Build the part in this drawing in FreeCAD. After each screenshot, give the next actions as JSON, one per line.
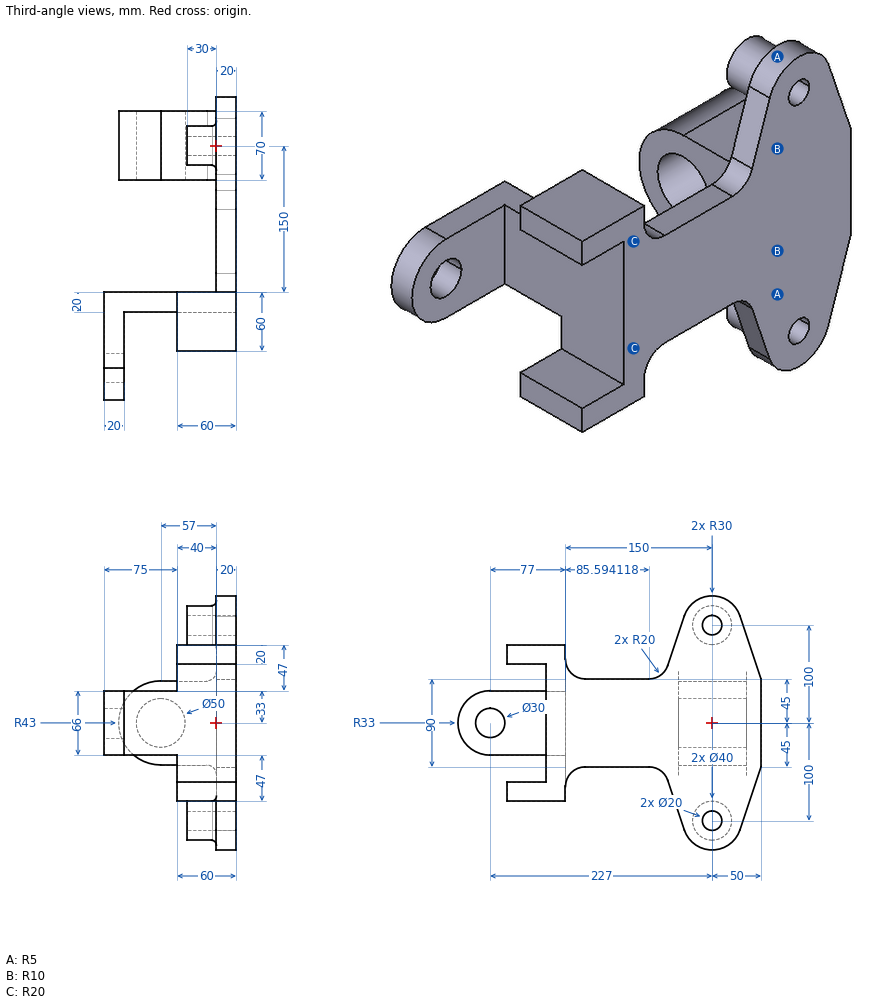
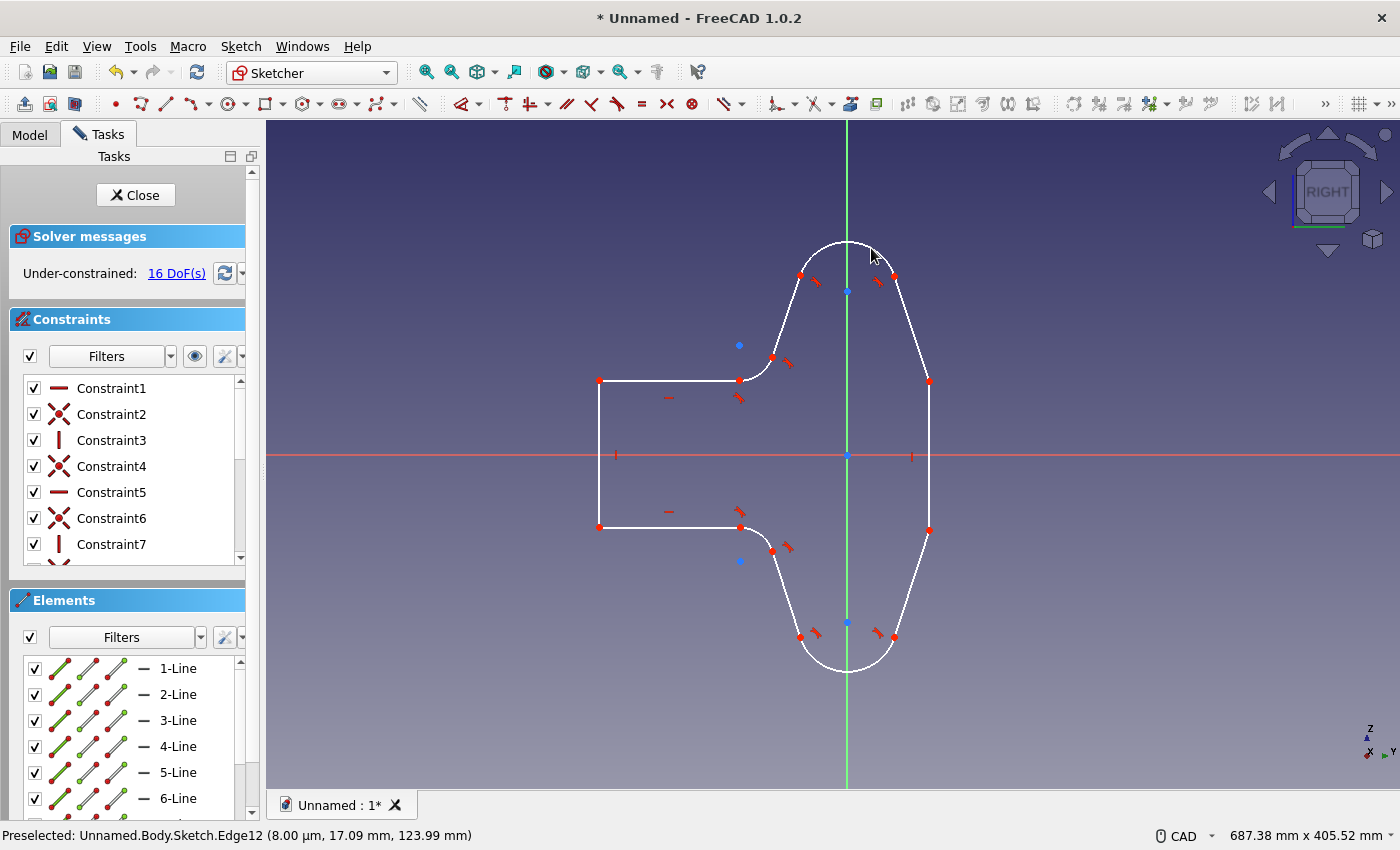
{"action": "left_click", "coordinate": [752, 378]}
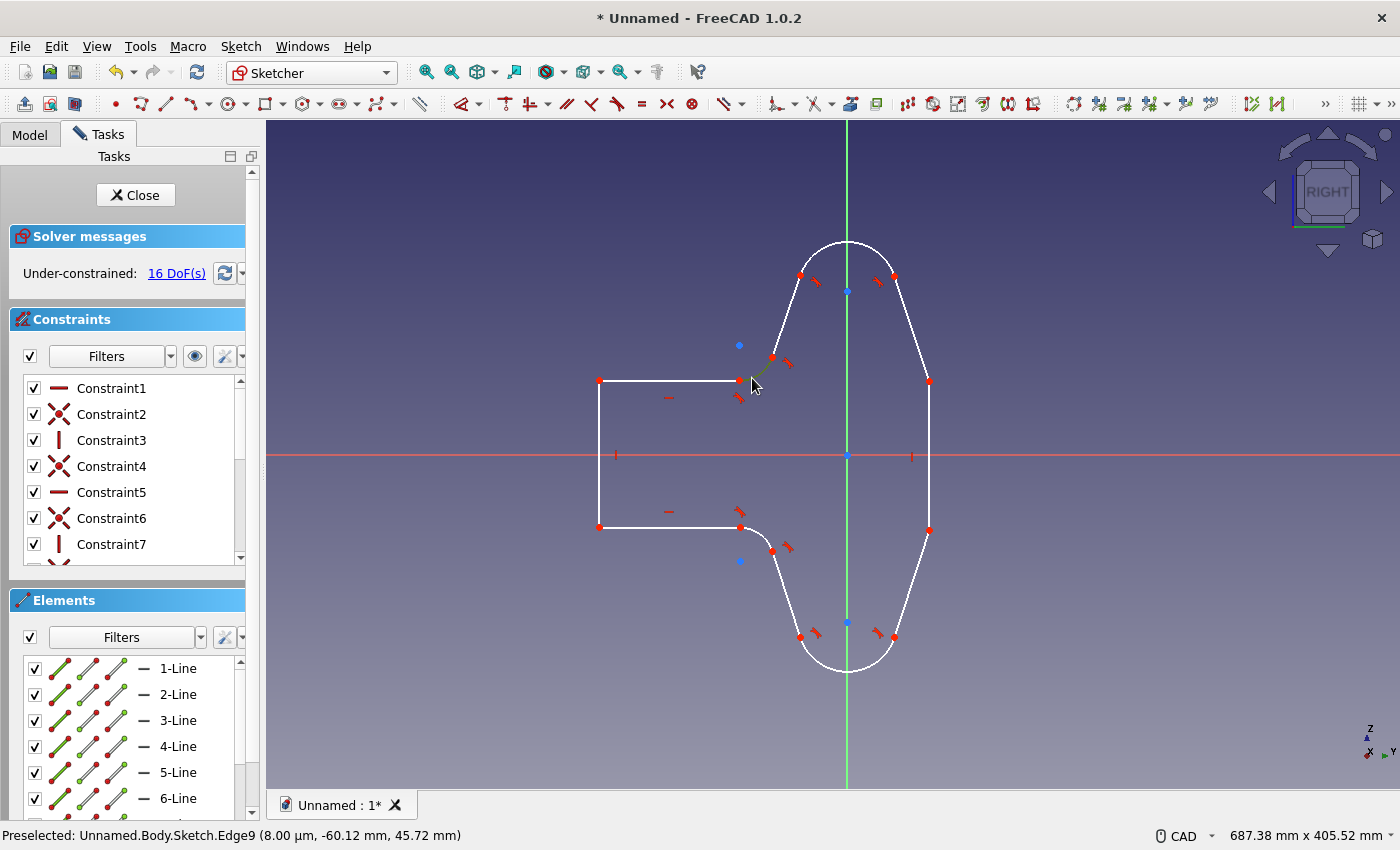
{"action": "left_click", "coordinate": [766, 540]}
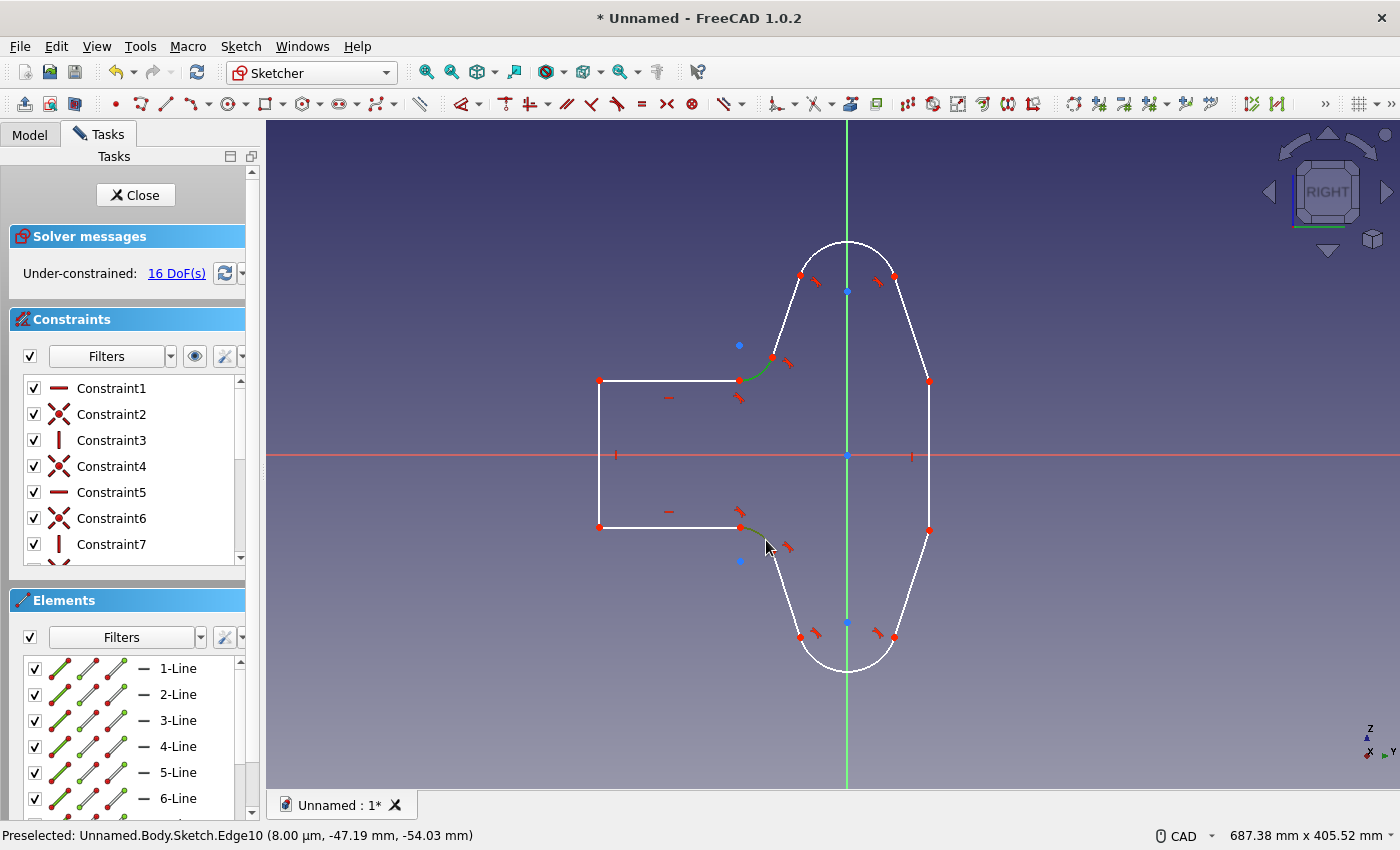
{"action": "left_click", "coordinate": [642, 104]}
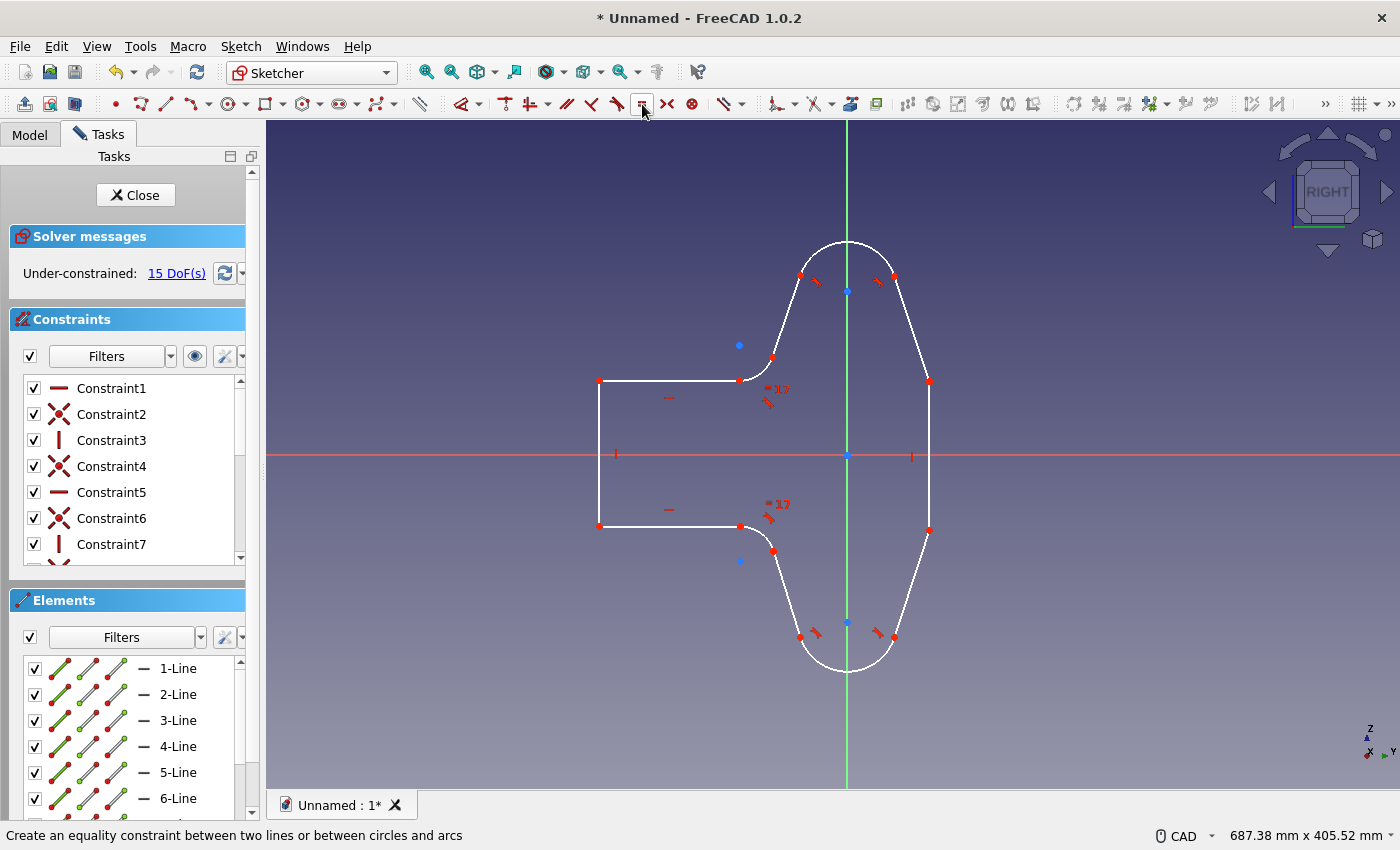
{"action": "left_click", "coordinate": [823, 665]}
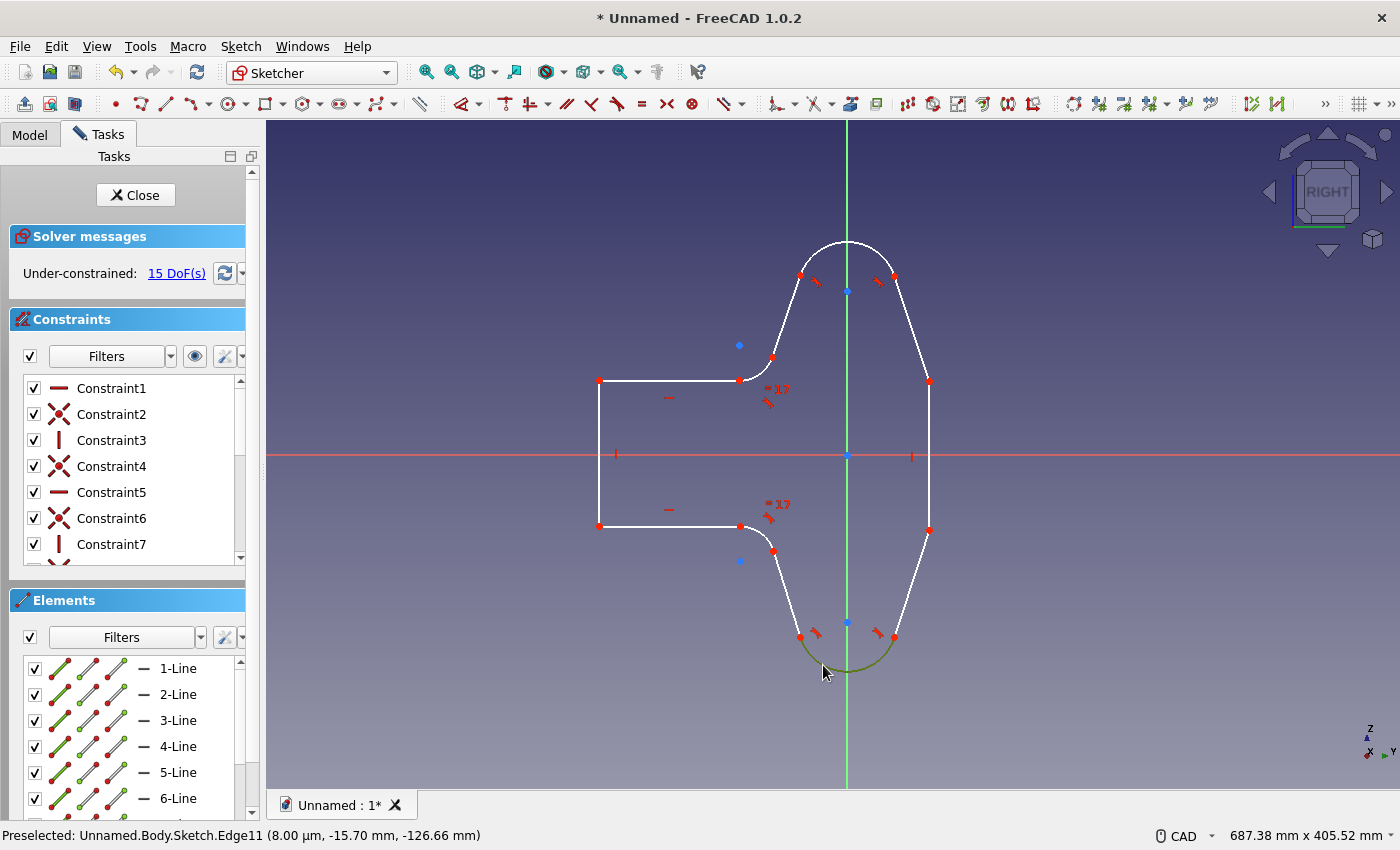
{"action": "left_click", "coordinate": [871, 248]}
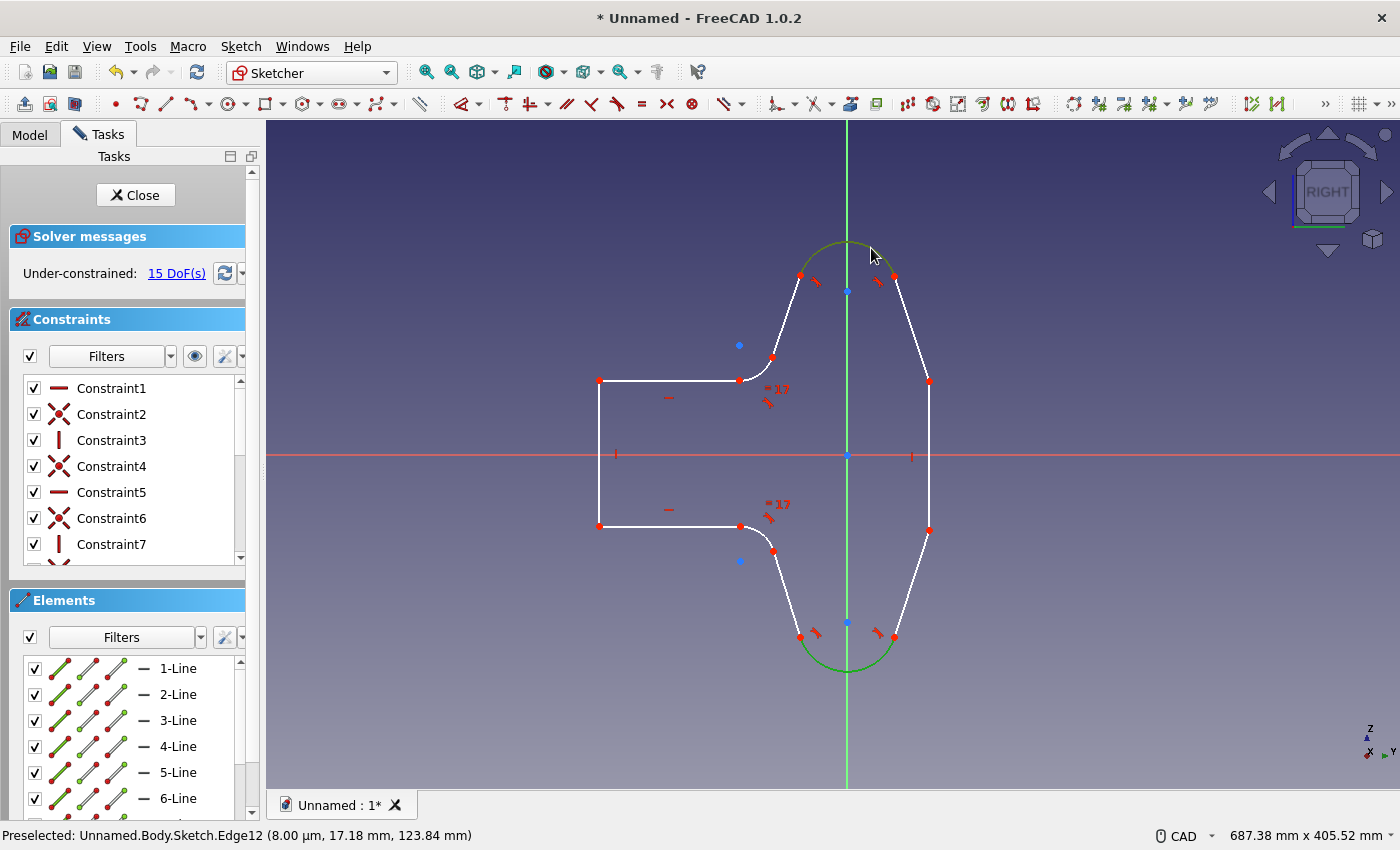
{"action": "left_click", "coordinate": [642, 104]}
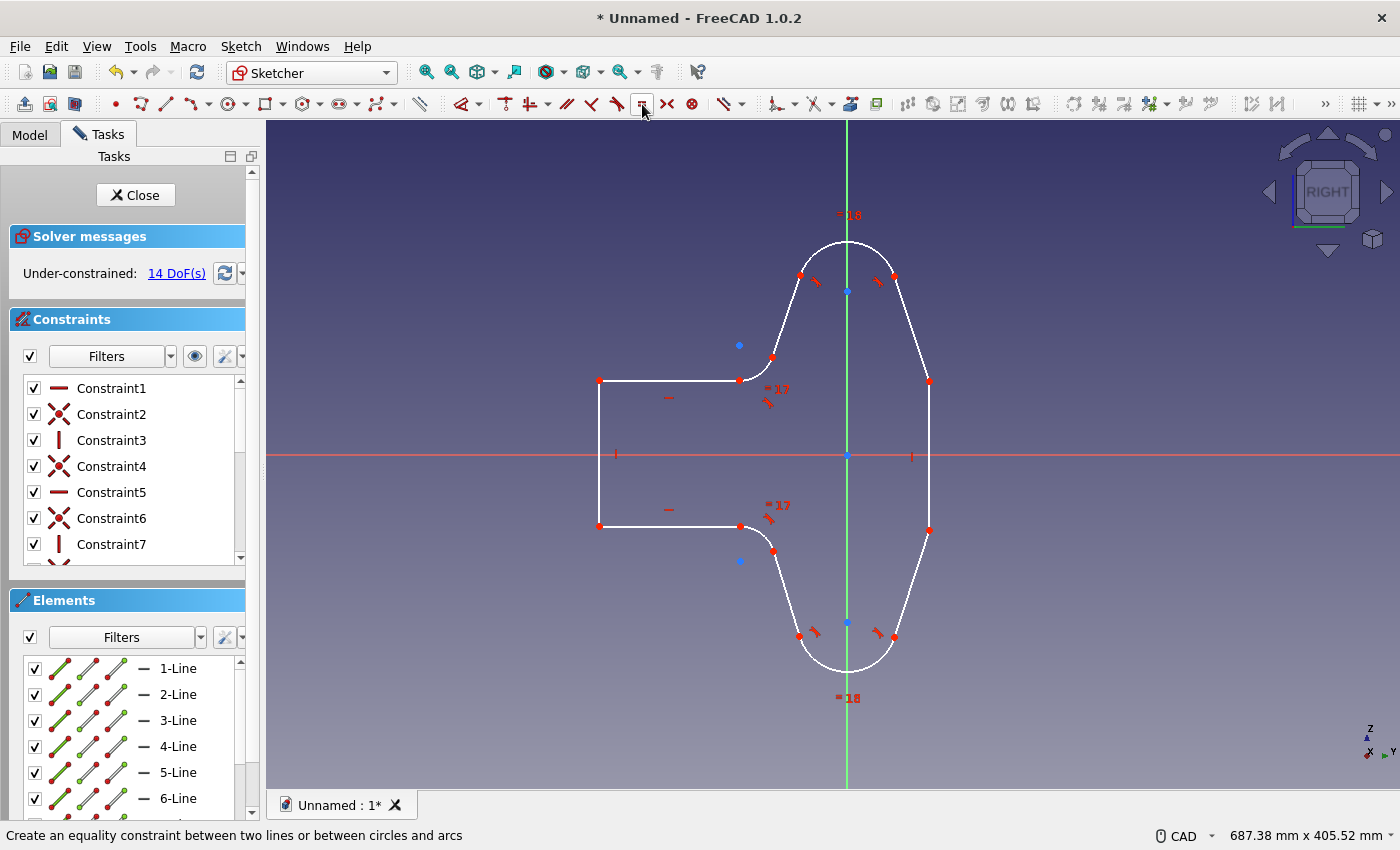
{"action": "left_click", "coordinate": [847, 622]}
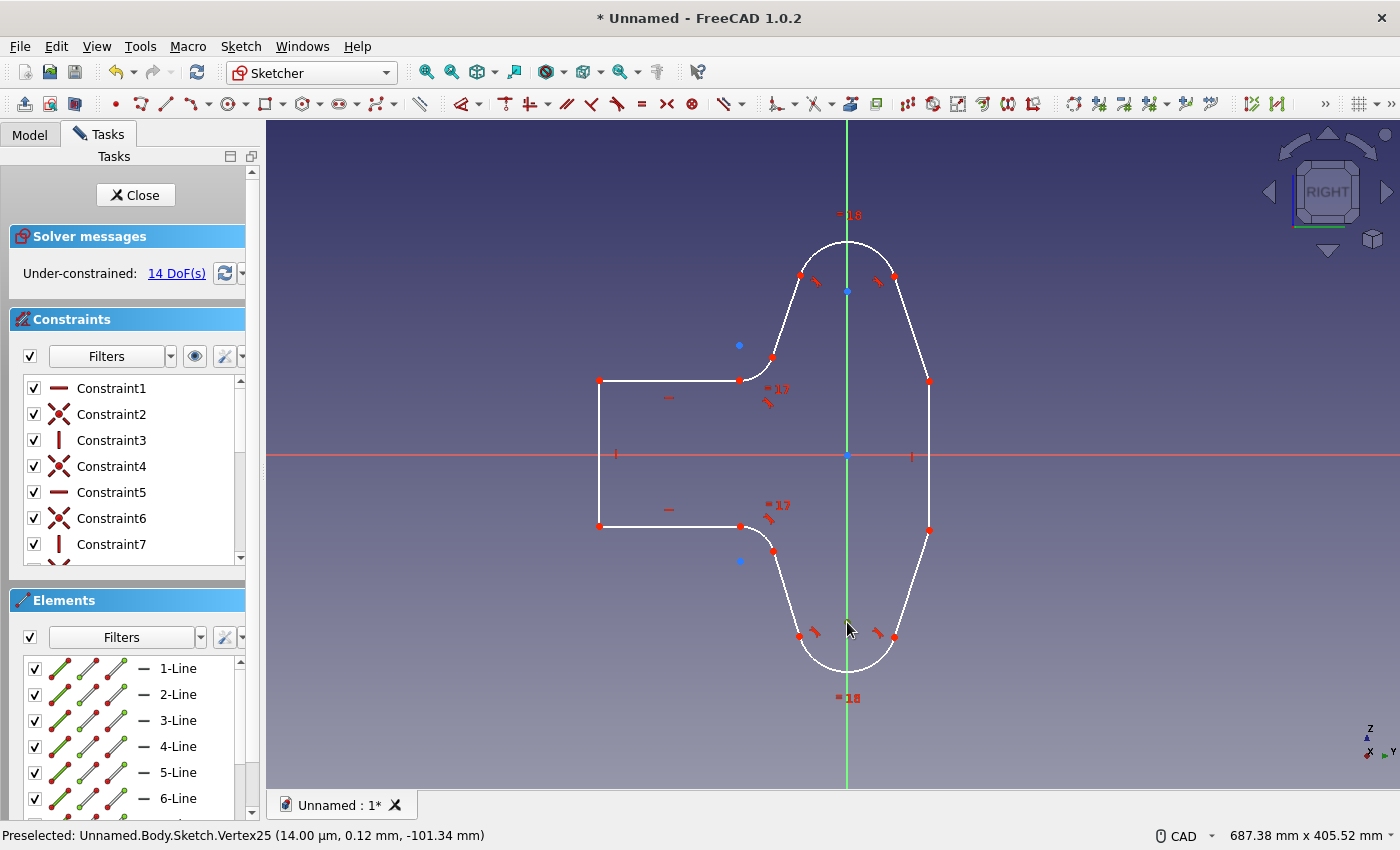
{"action": "left_click", "coordinate": [847, 717]}